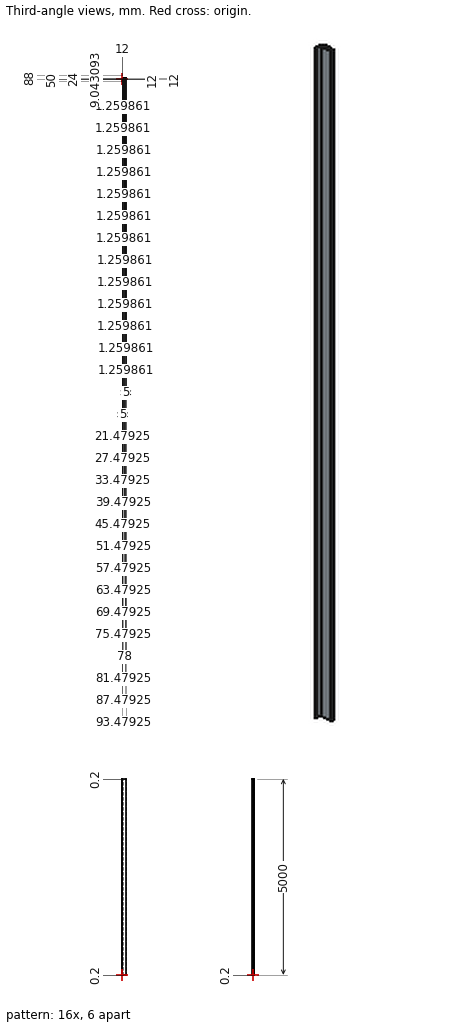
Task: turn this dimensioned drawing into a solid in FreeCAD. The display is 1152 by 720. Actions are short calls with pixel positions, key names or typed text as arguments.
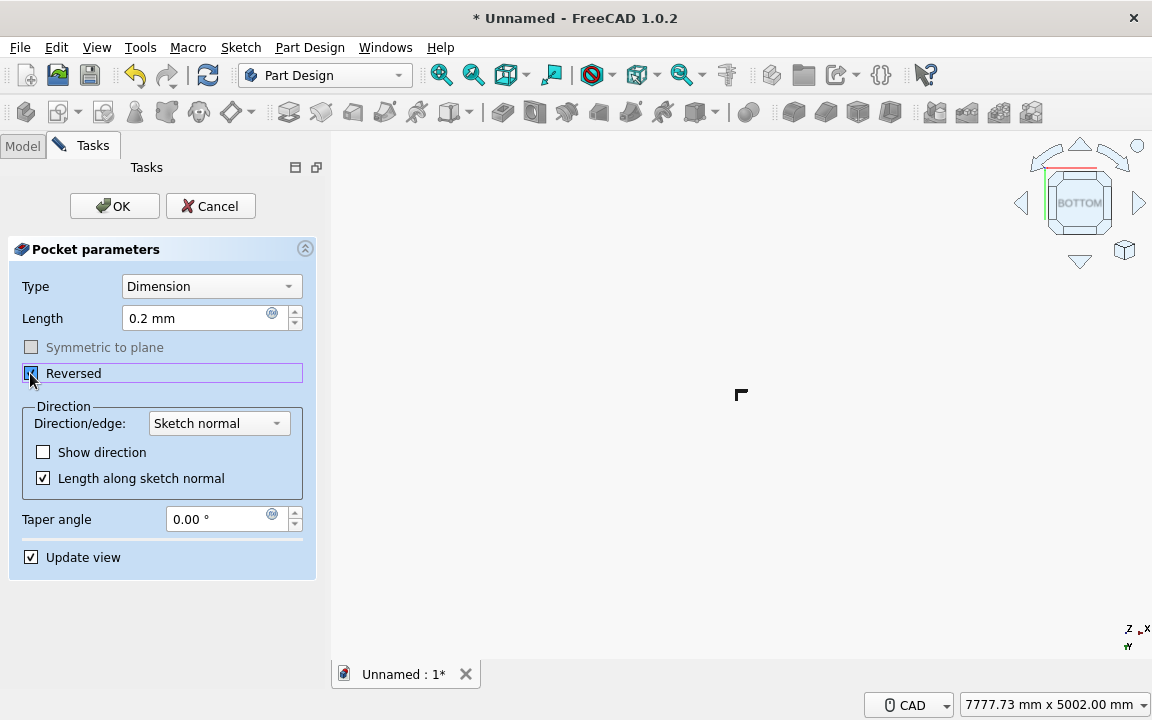
click(115, 206)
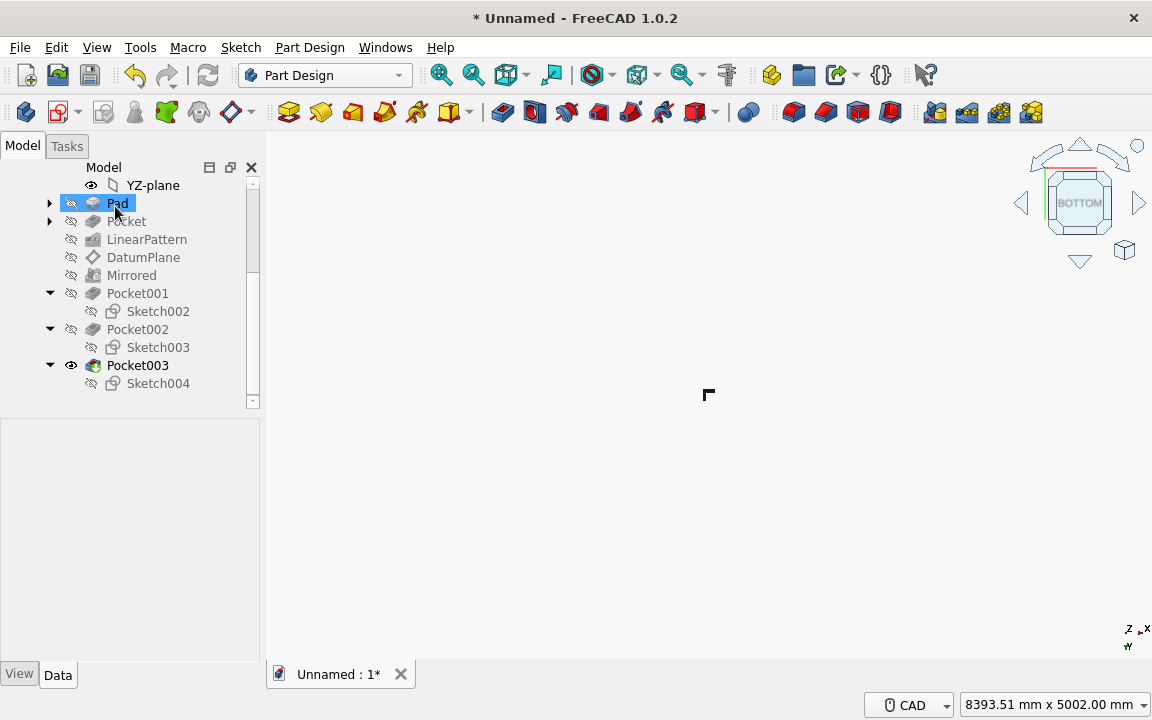
click(442, 76)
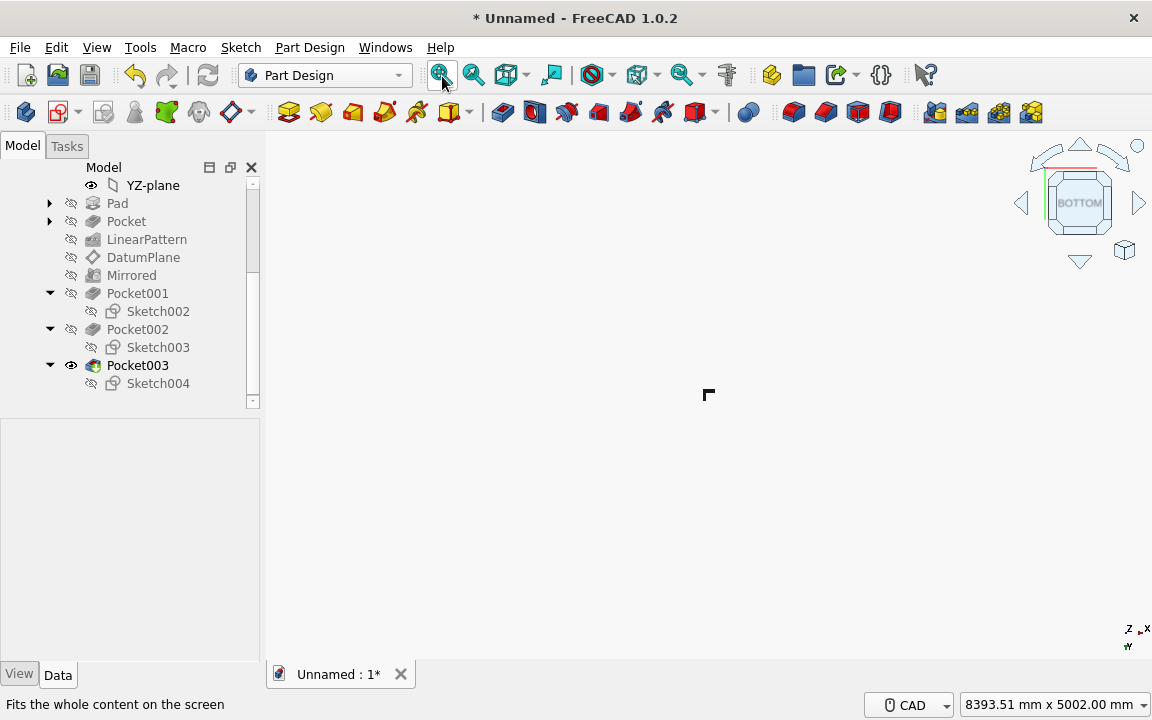
click(58, 112)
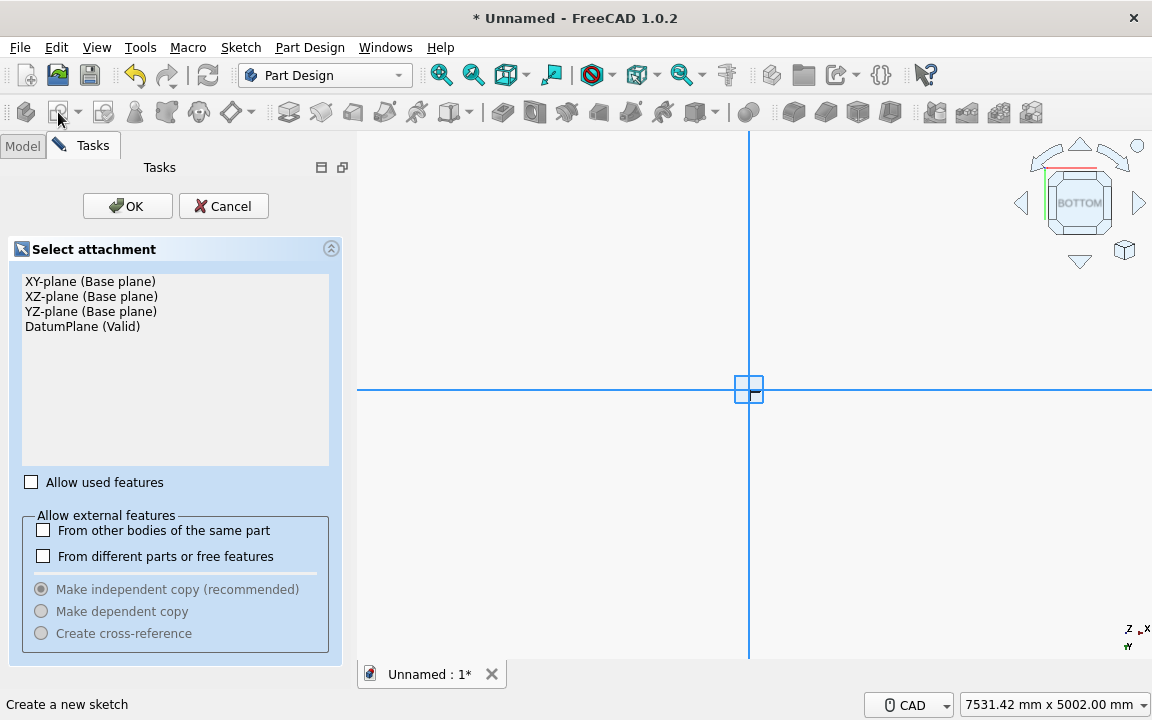
click(82, 282)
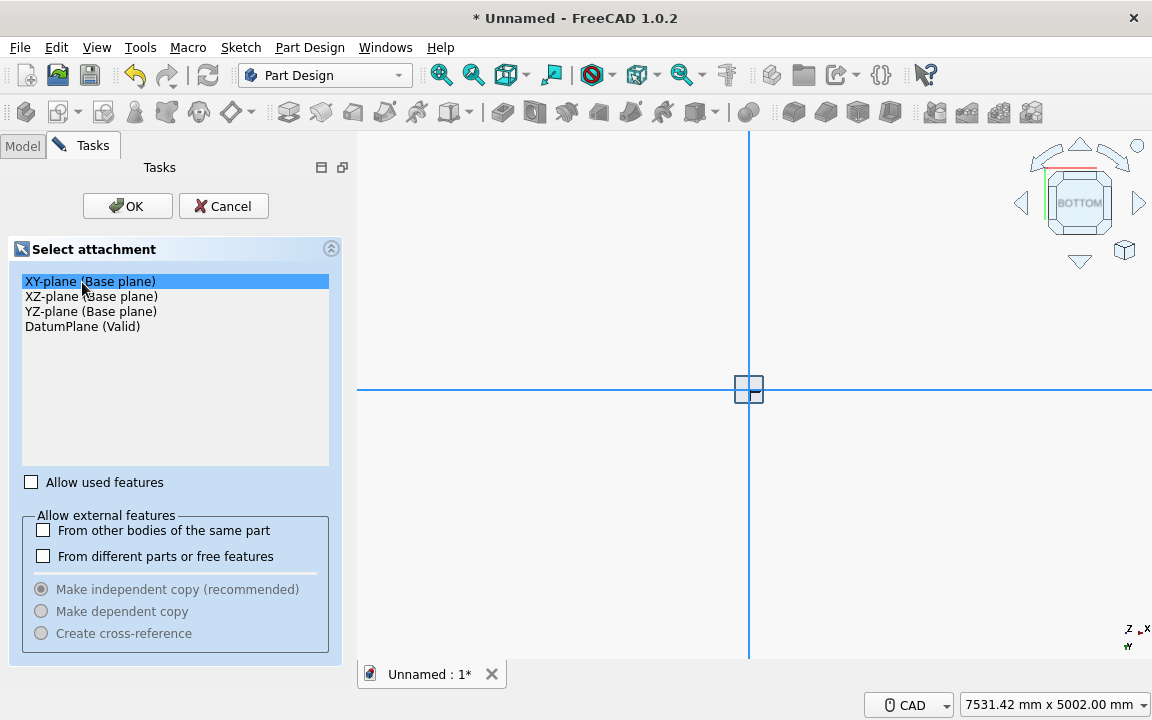
click(128, 206)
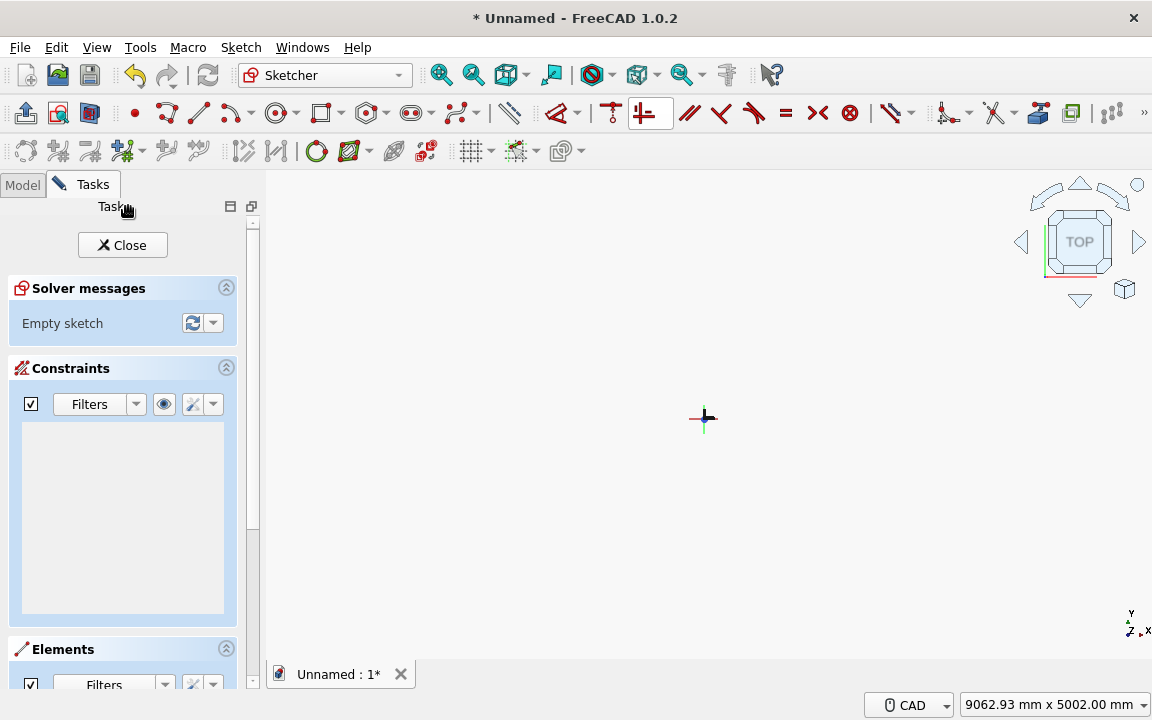
key(q)
key(s)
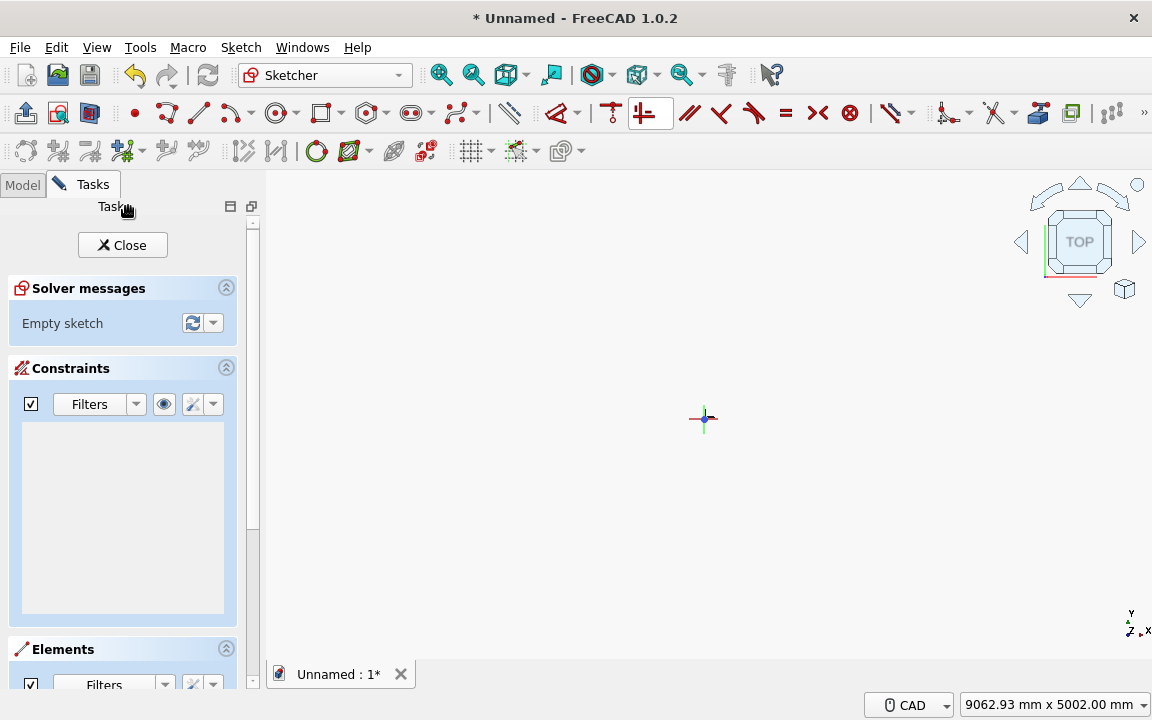
scroll(712, 418, up, 15)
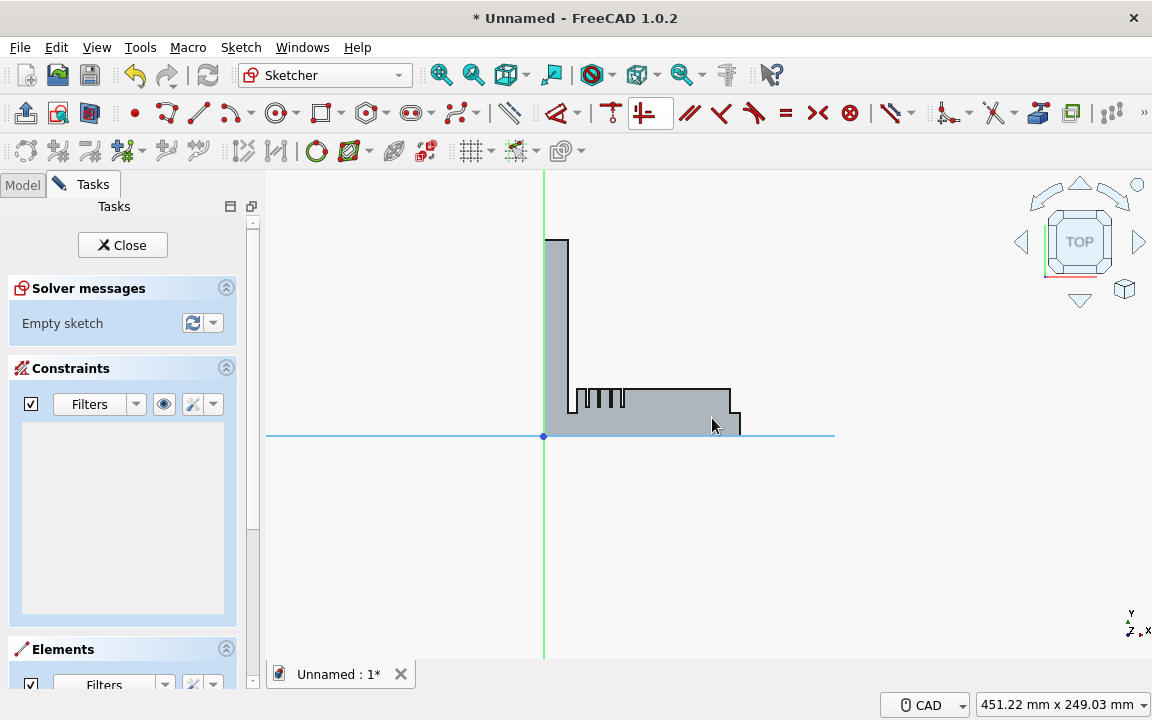
scroll(634, 397, up, 14)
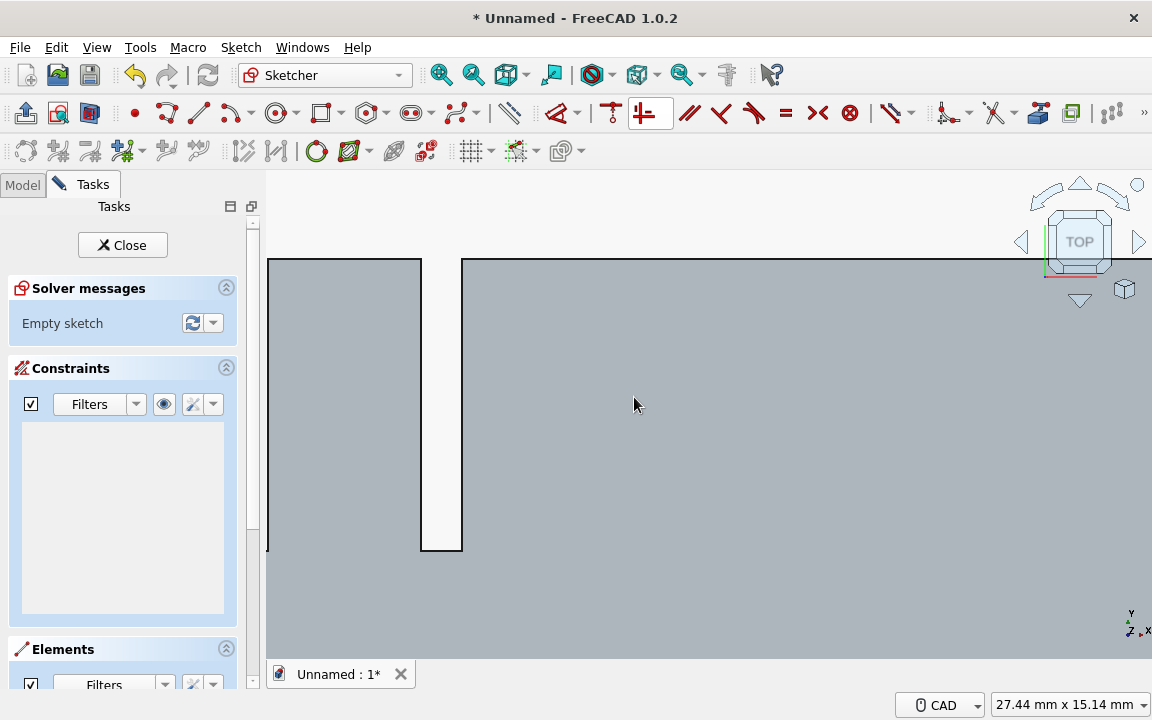
click(322, 114)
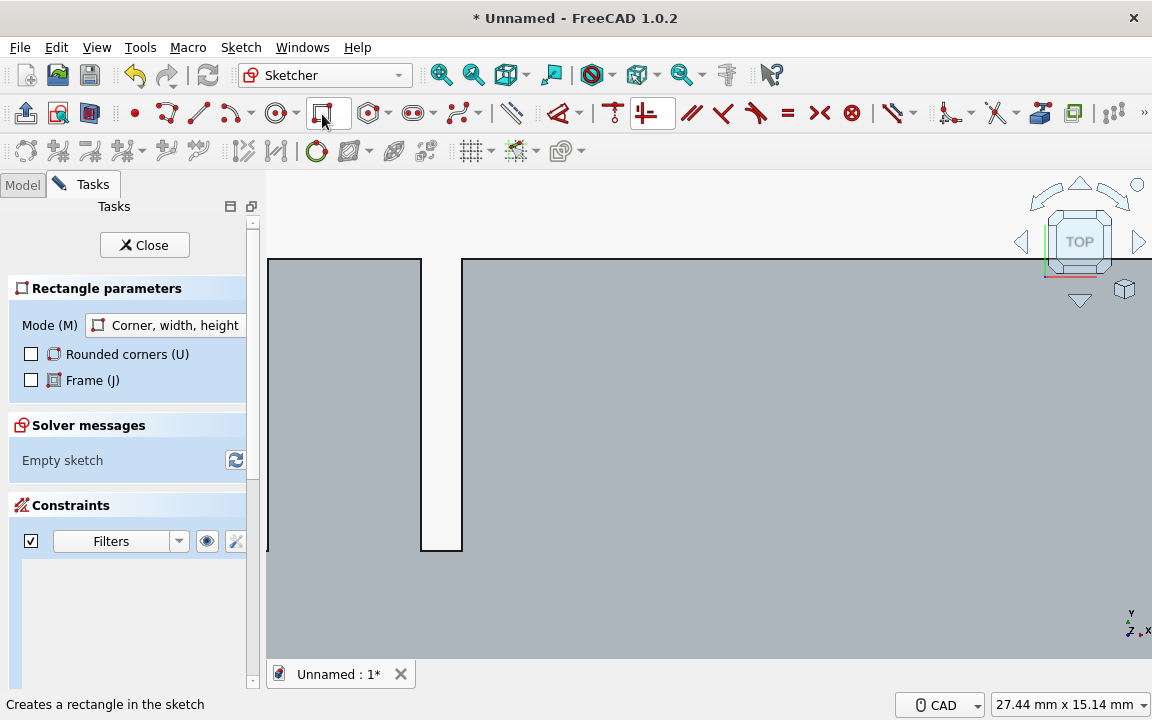
click(615, 259)
click(656, 551)
key(Escape)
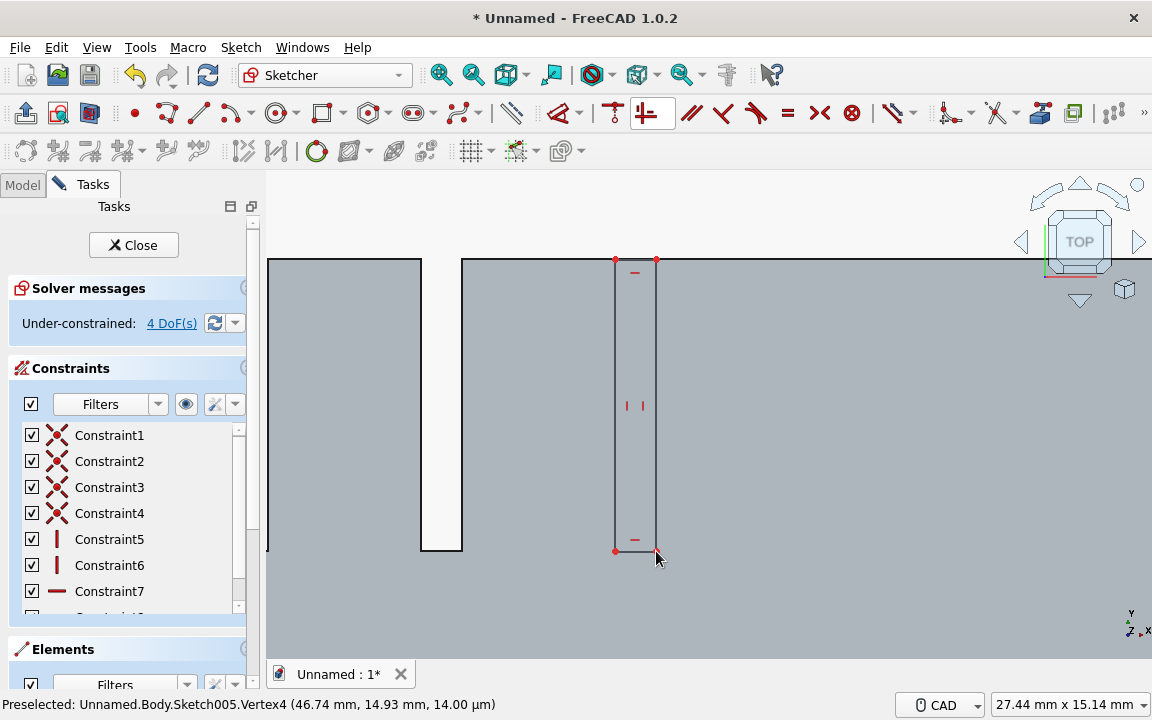
click(558, 114)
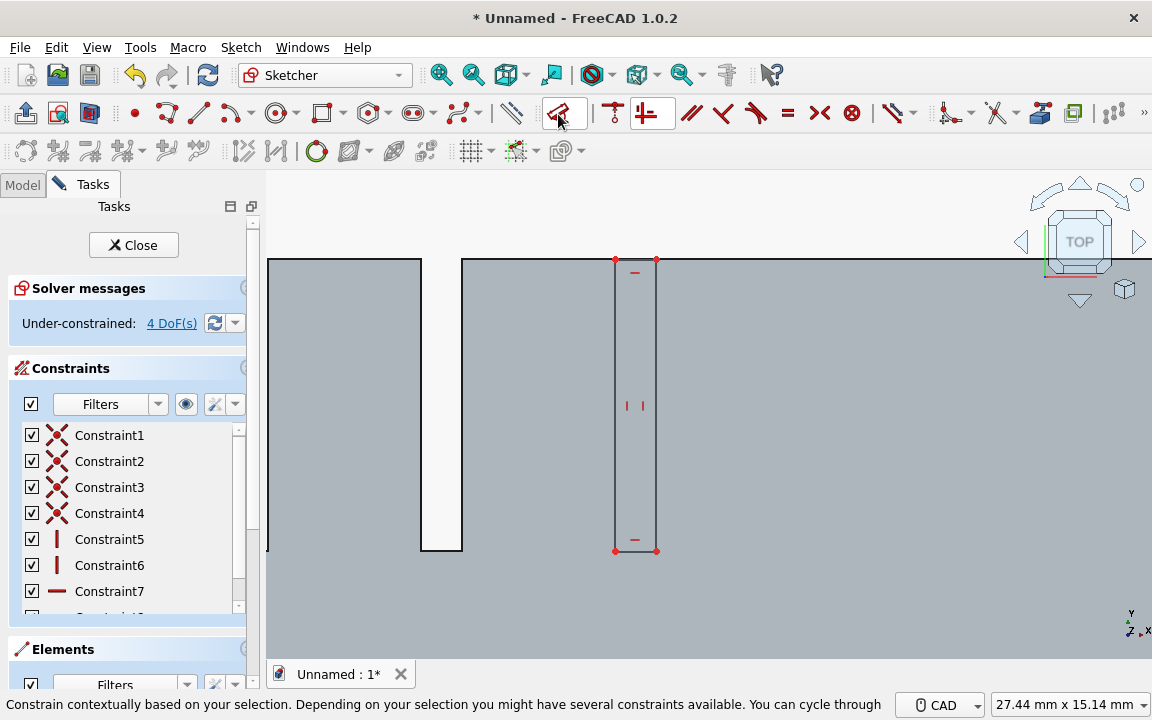
click(615, 260)
click(649, 575)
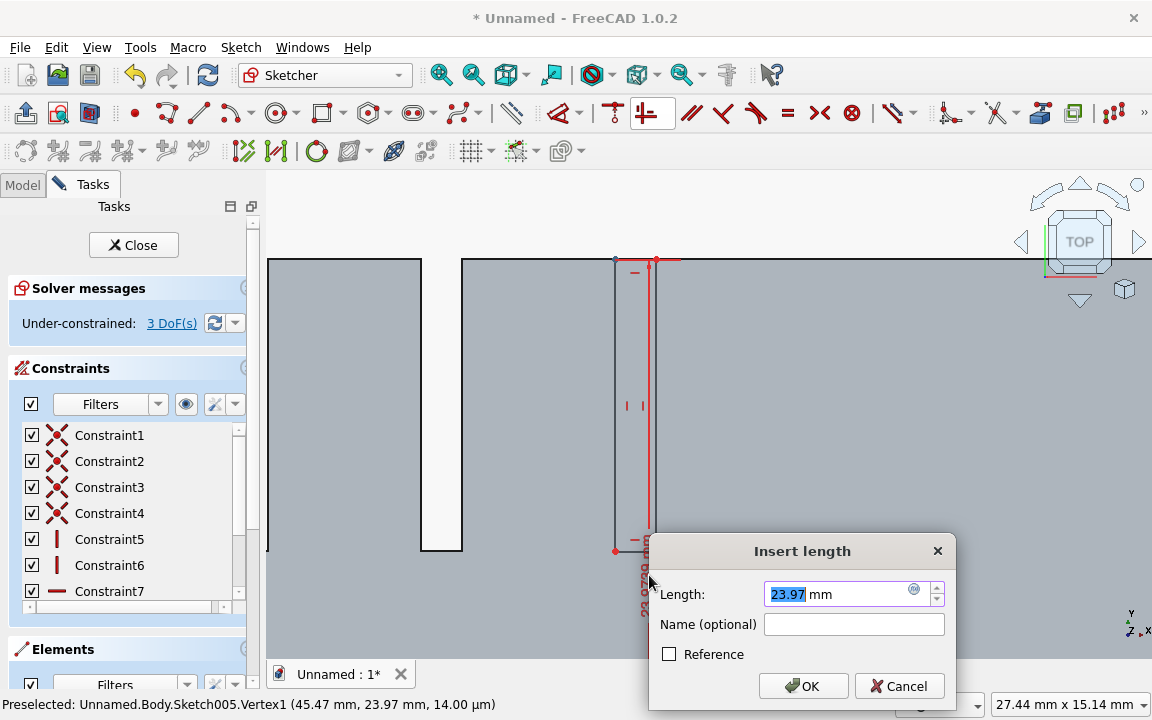
text(24)
key(Return)